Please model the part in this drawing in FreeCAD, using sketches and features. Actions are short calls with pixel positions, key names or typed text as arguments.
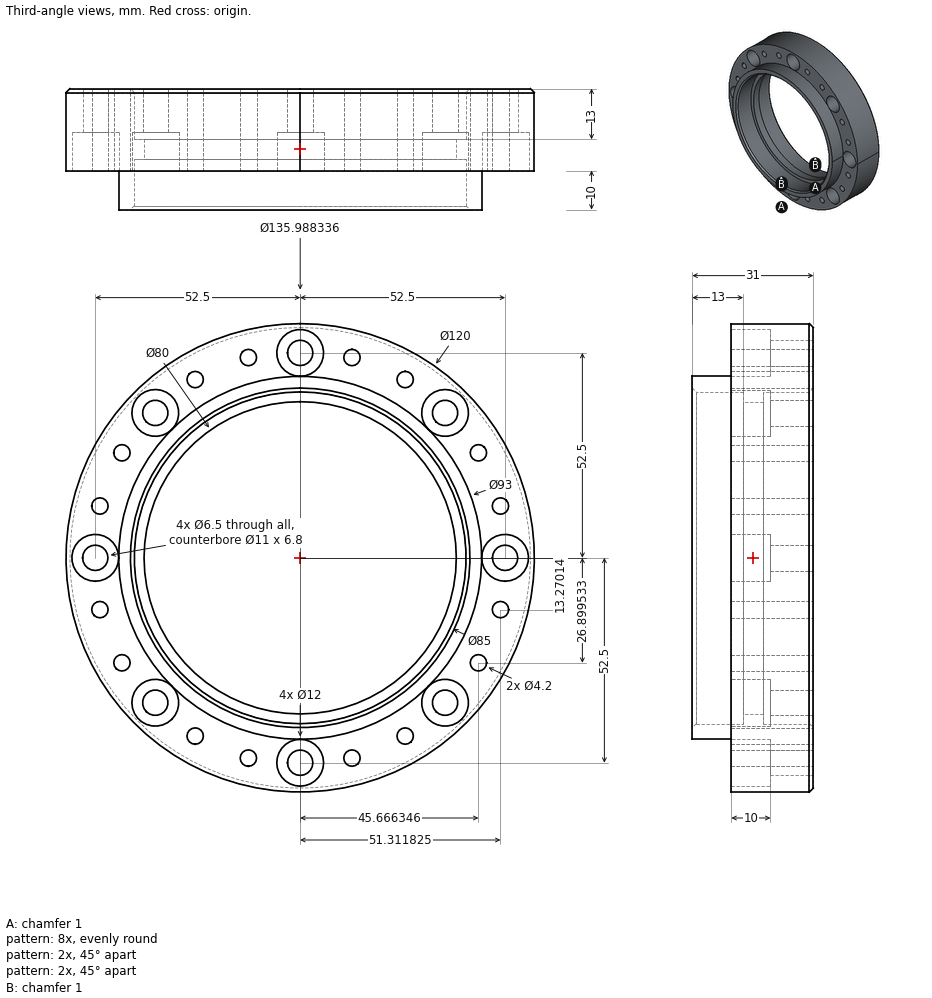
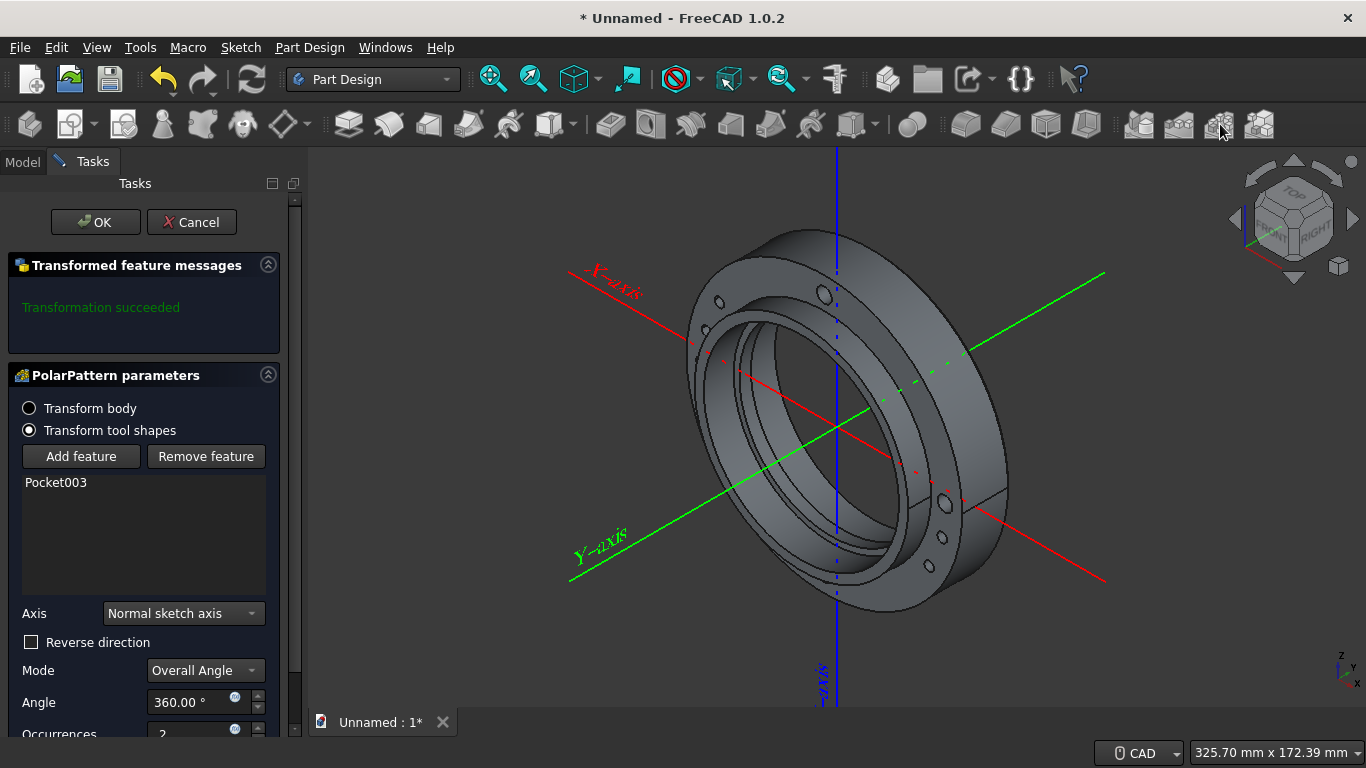
click(184, 614)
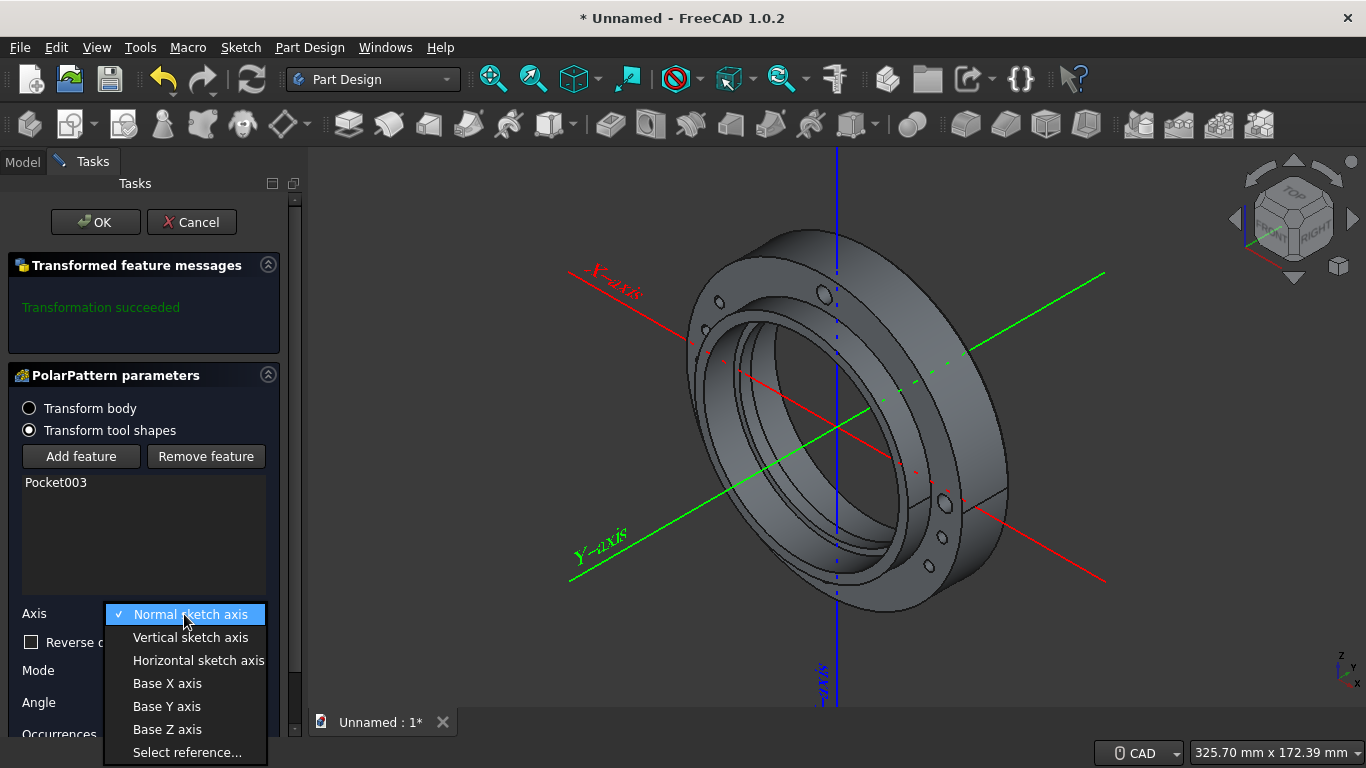
click(184, 706)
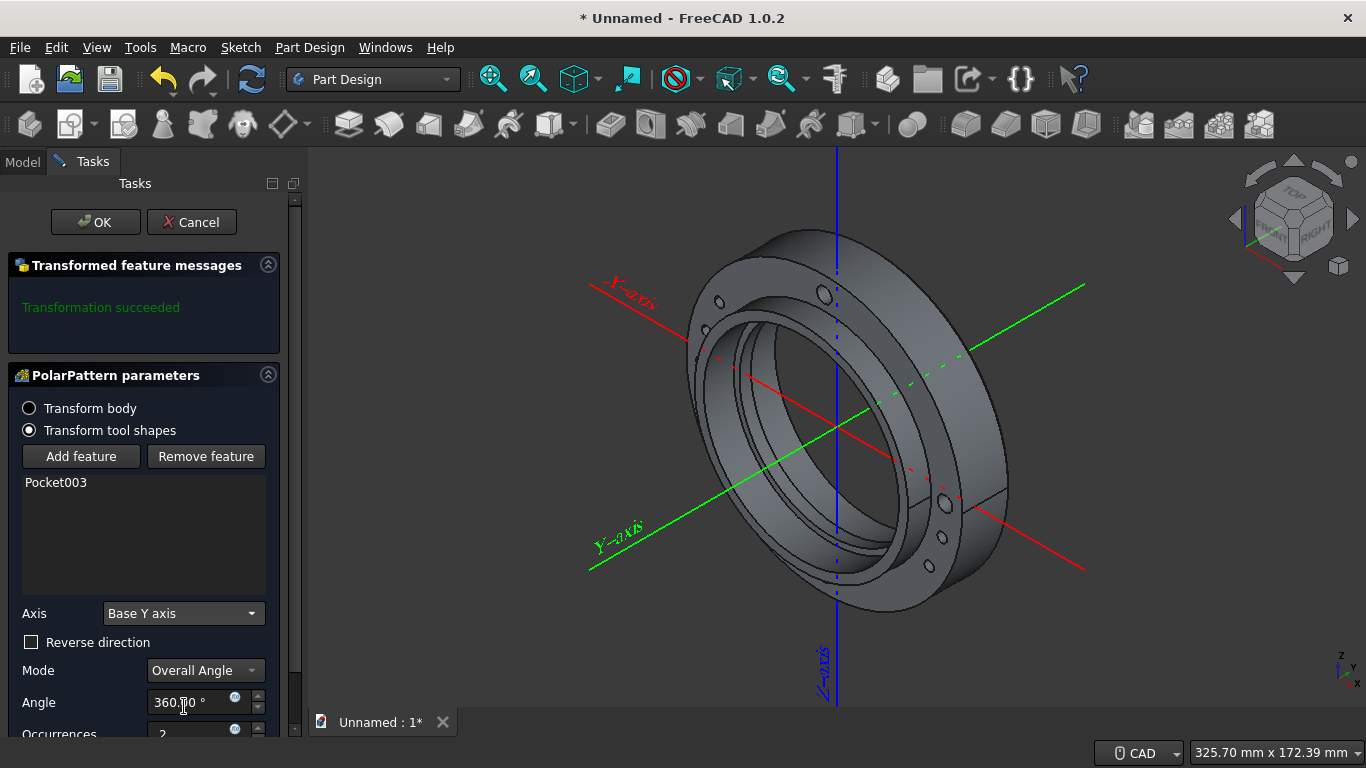
scroll(295, 464, down, 2)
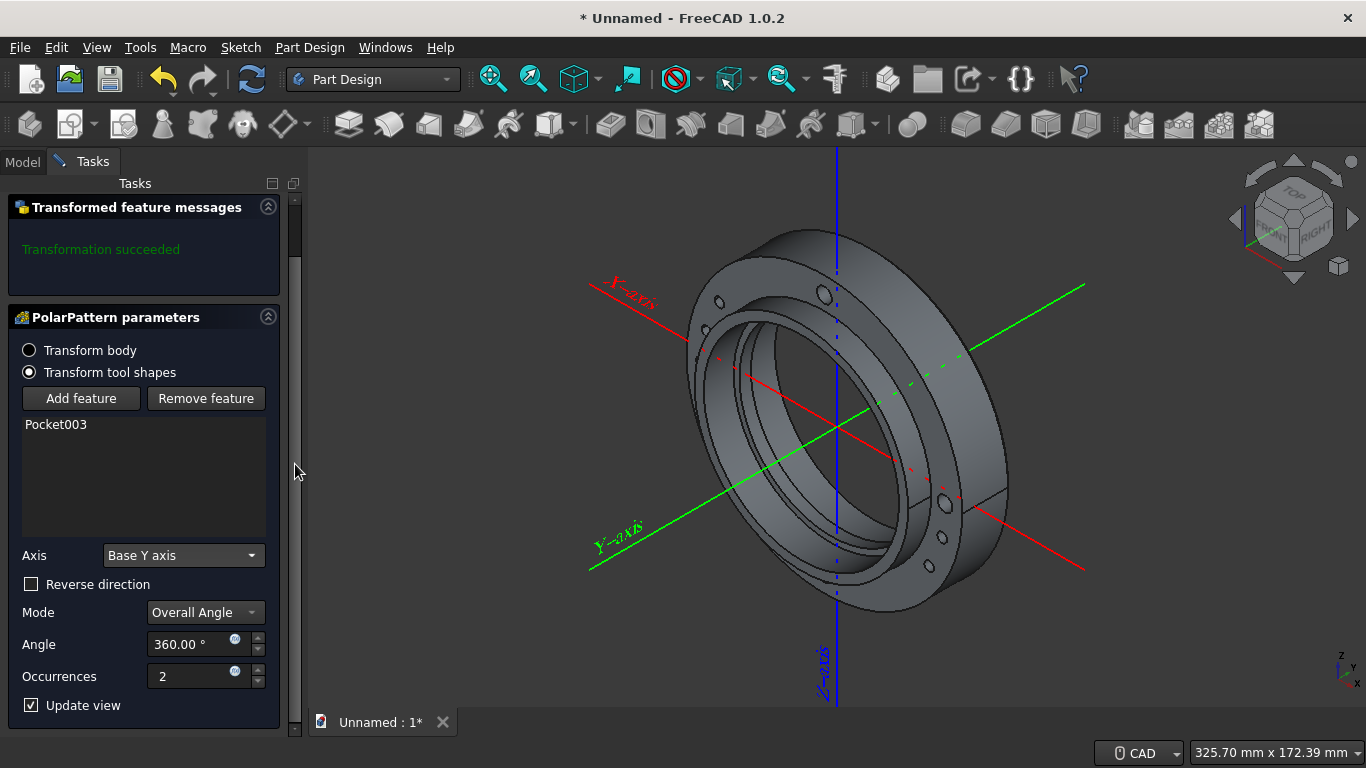
triple_click(198, 676)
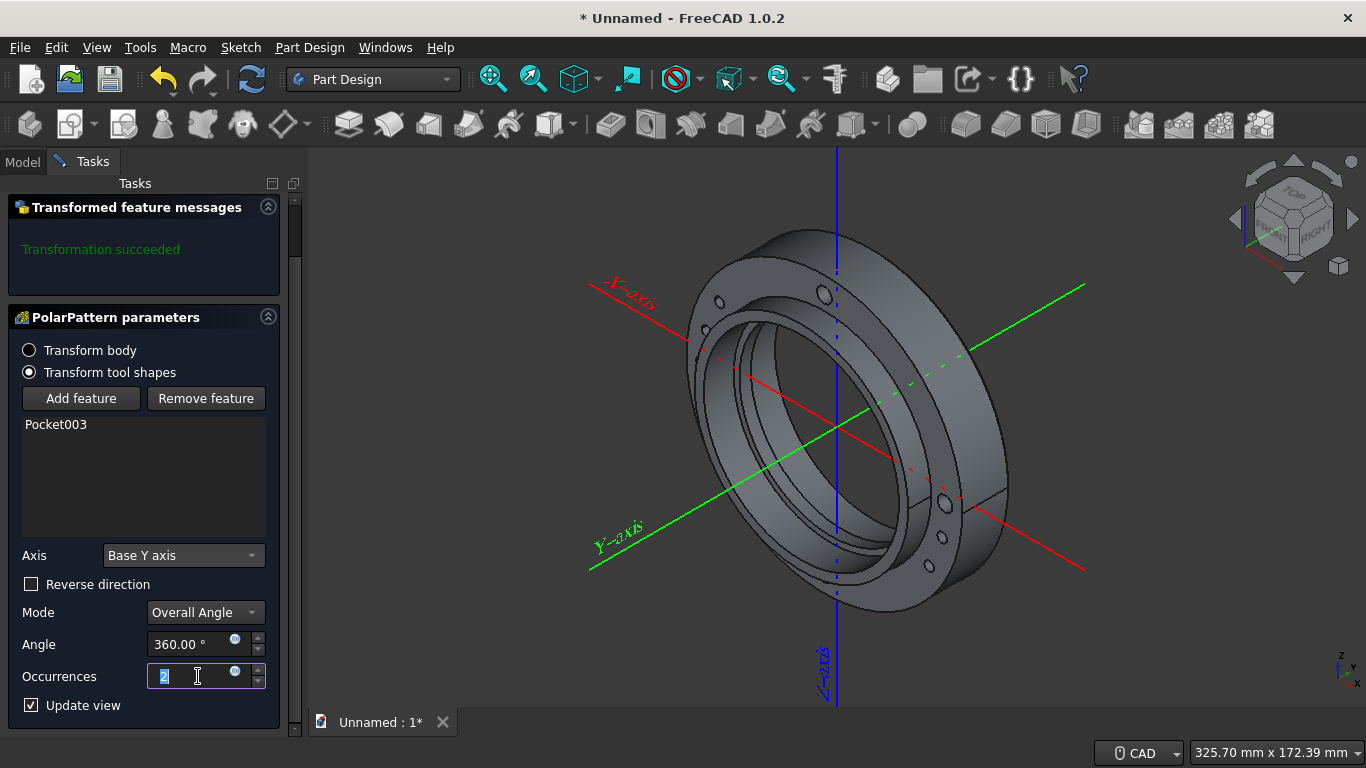
text(8)
key(Tab)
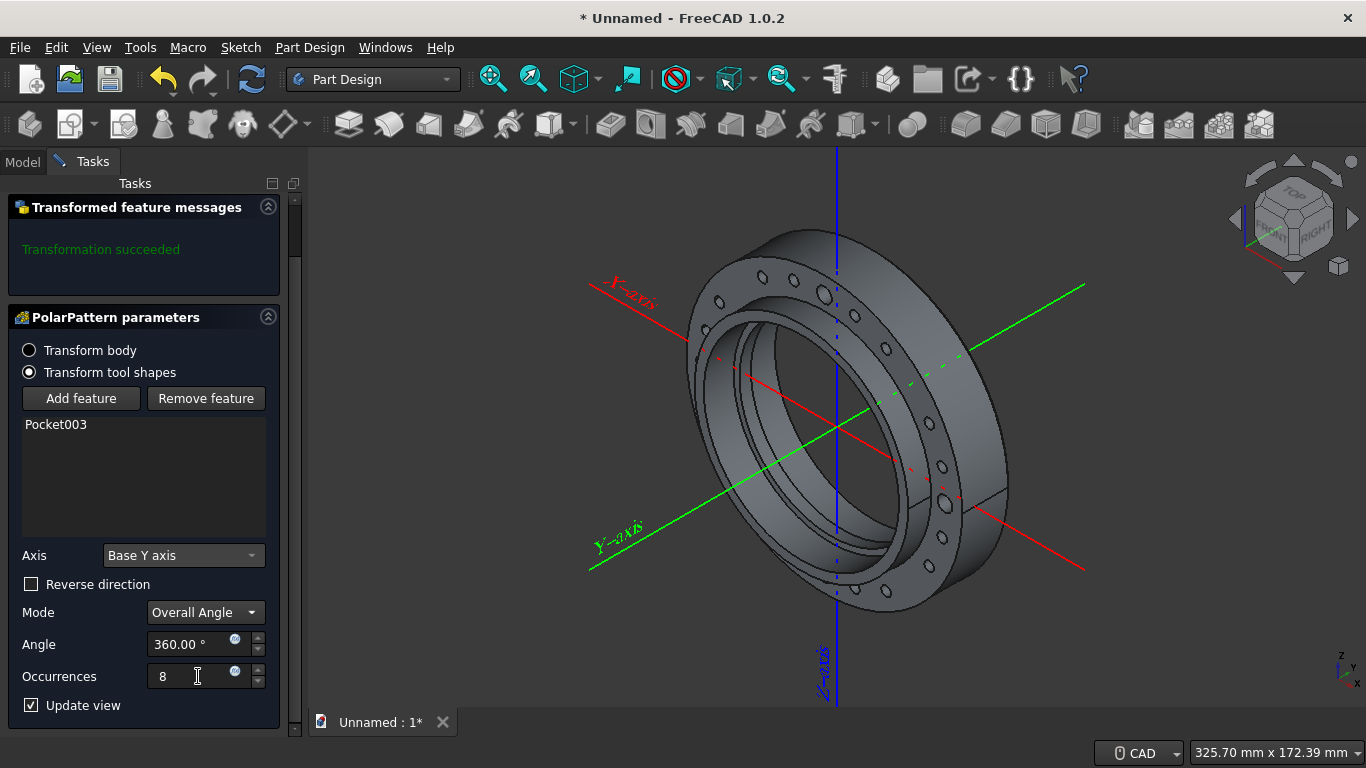
scroll(295, 464, up, 2)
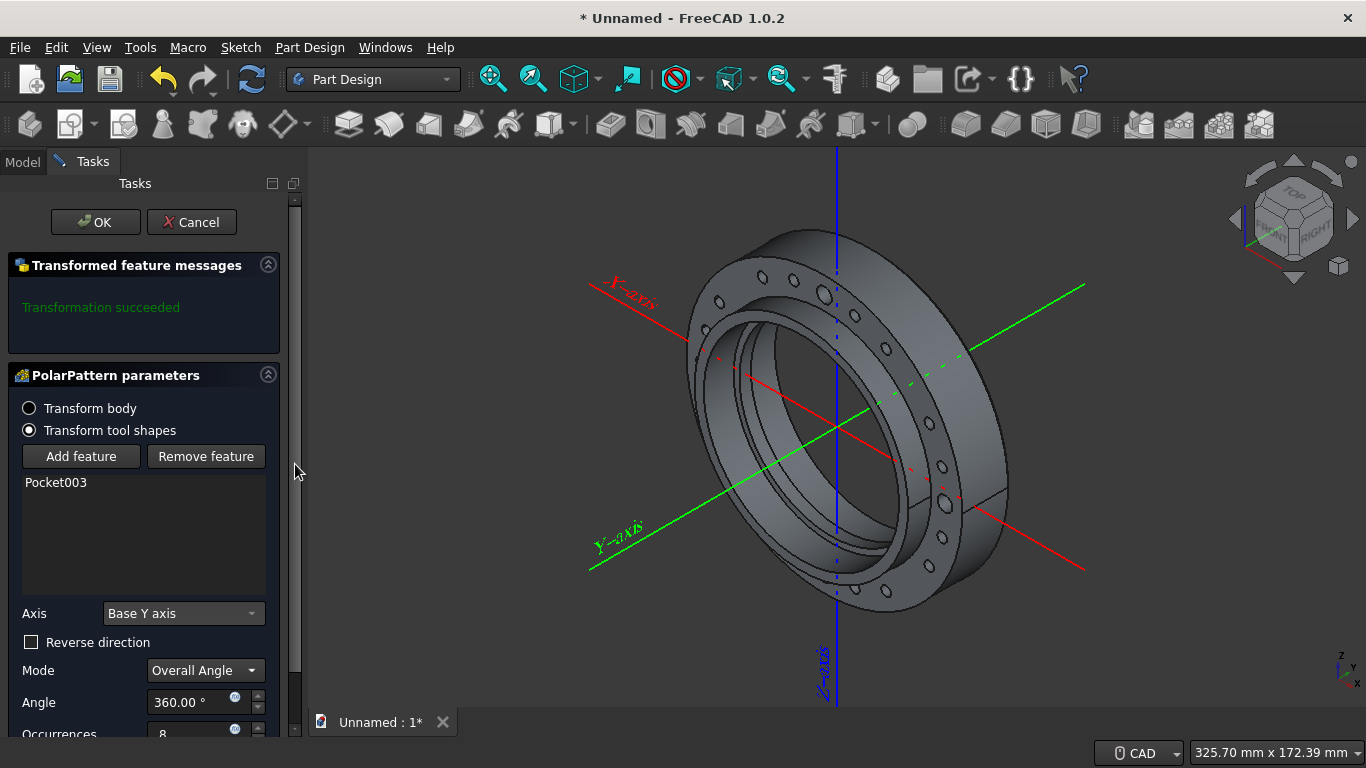
click(96, 222)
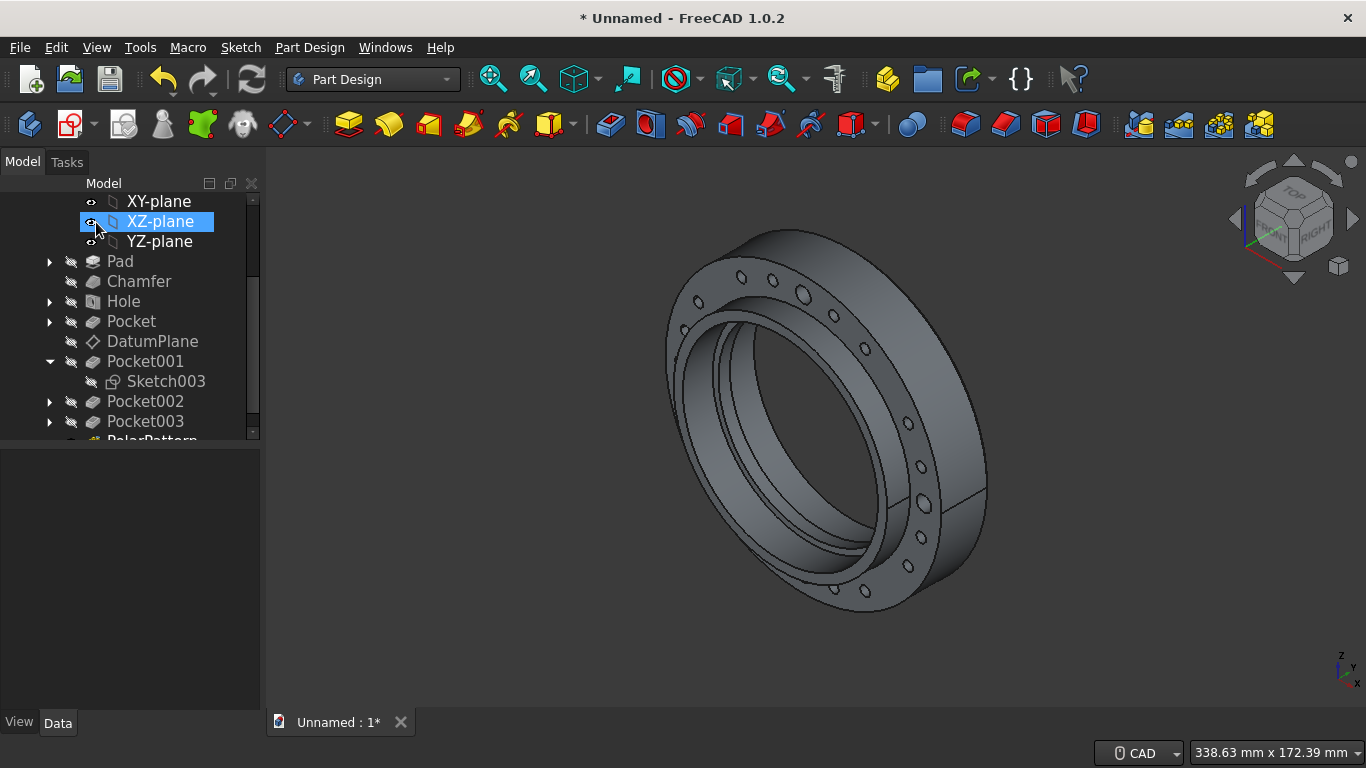
click(725, 297)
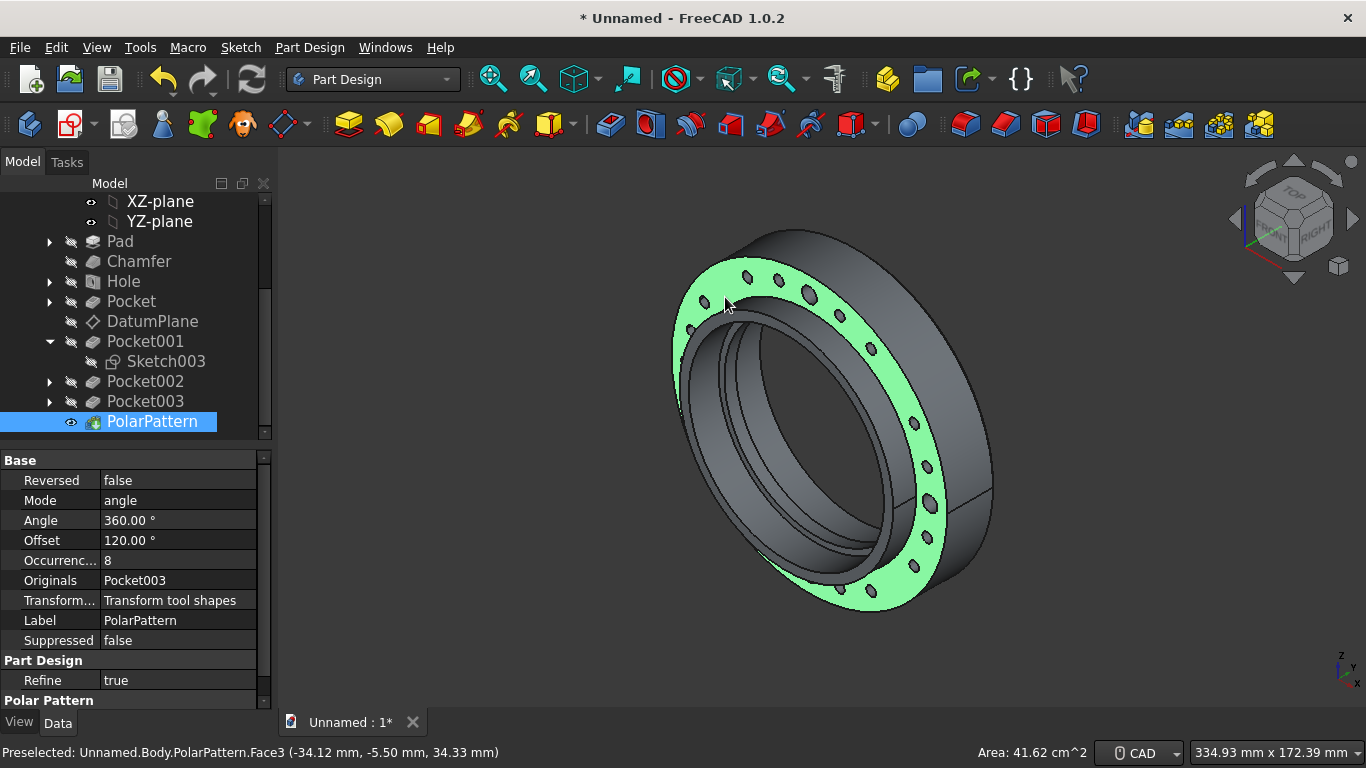
click(70, 124)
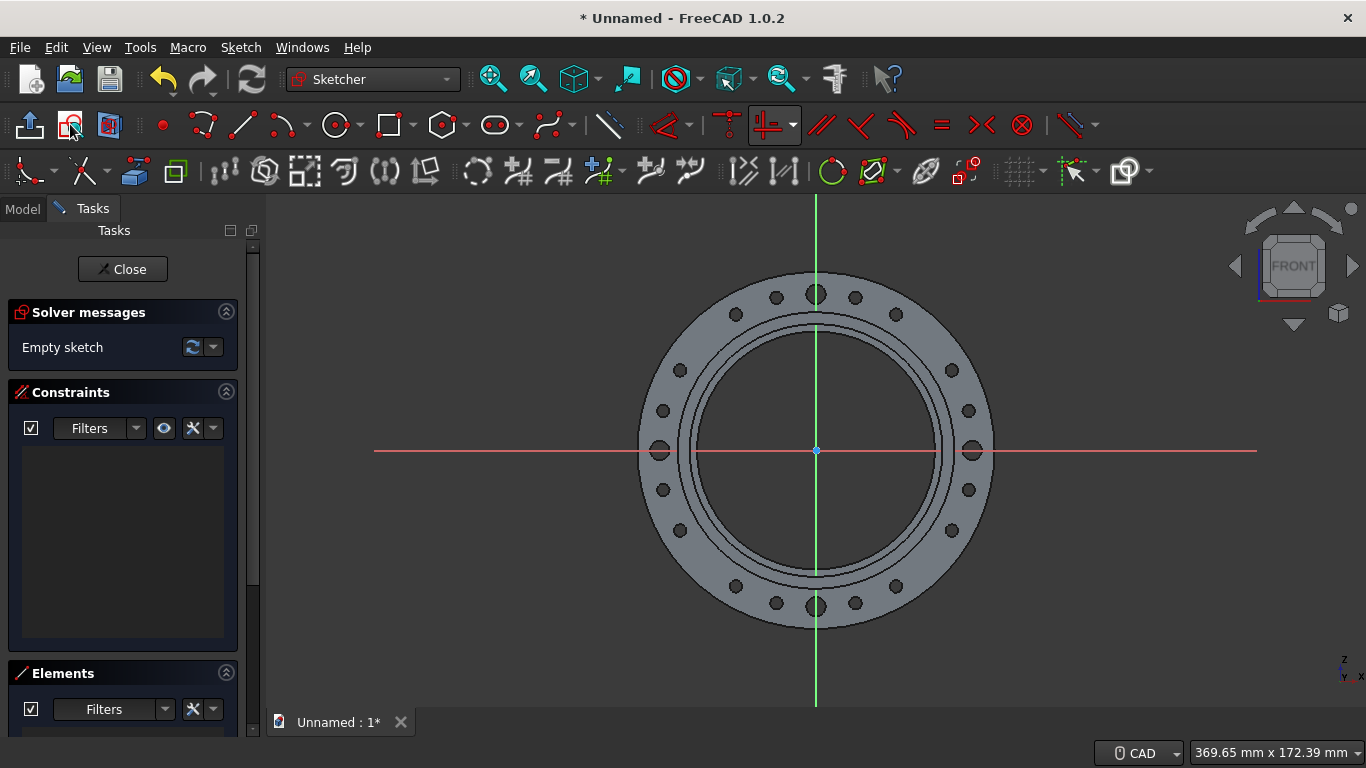
click(336, 126)